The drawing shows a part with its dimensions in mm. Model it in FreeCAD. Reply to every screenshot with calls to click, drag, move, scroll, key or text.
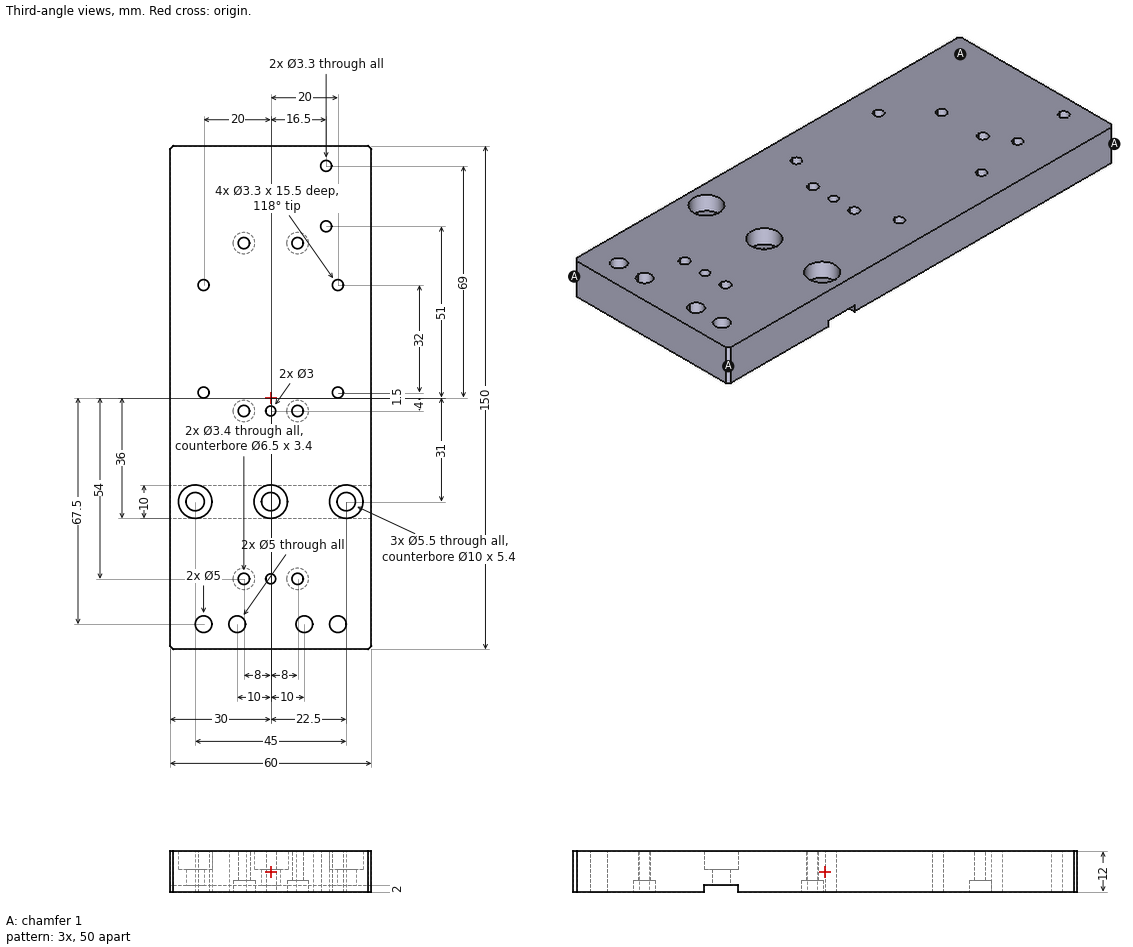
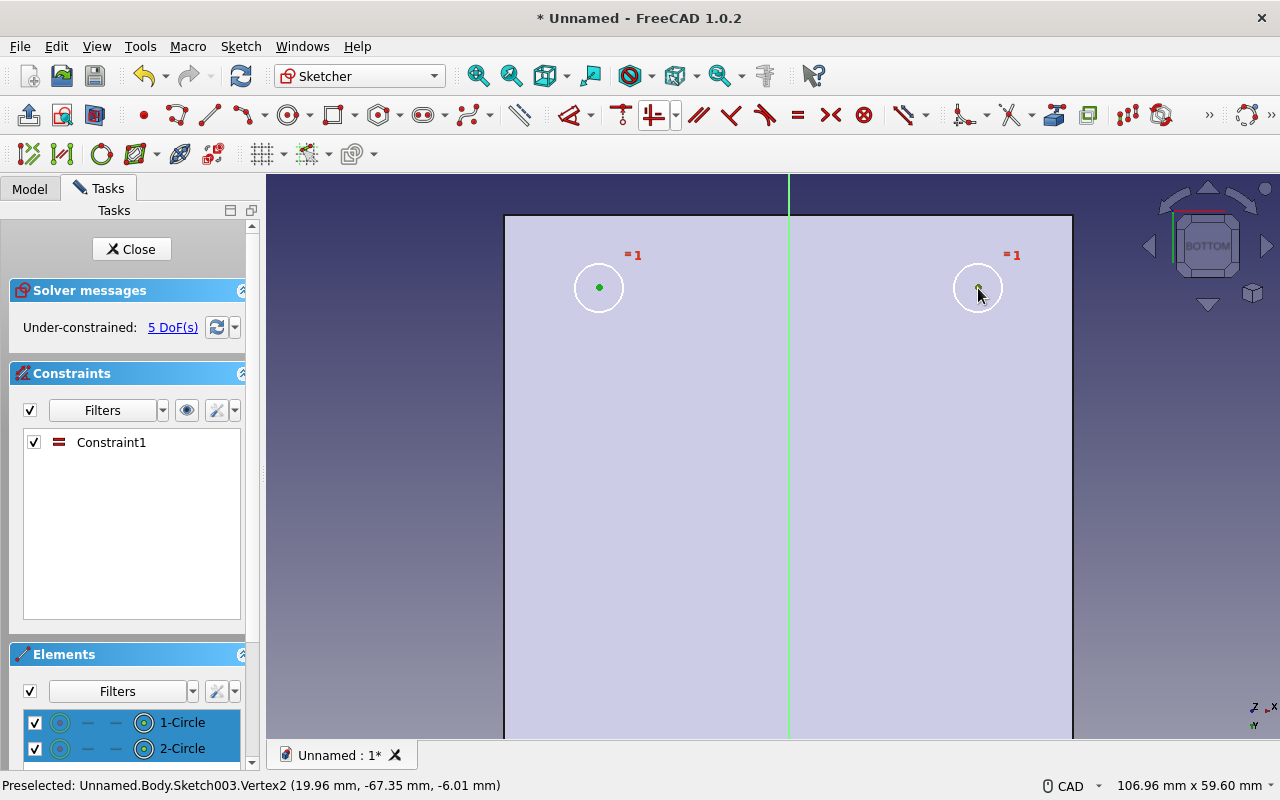
click(676, 116)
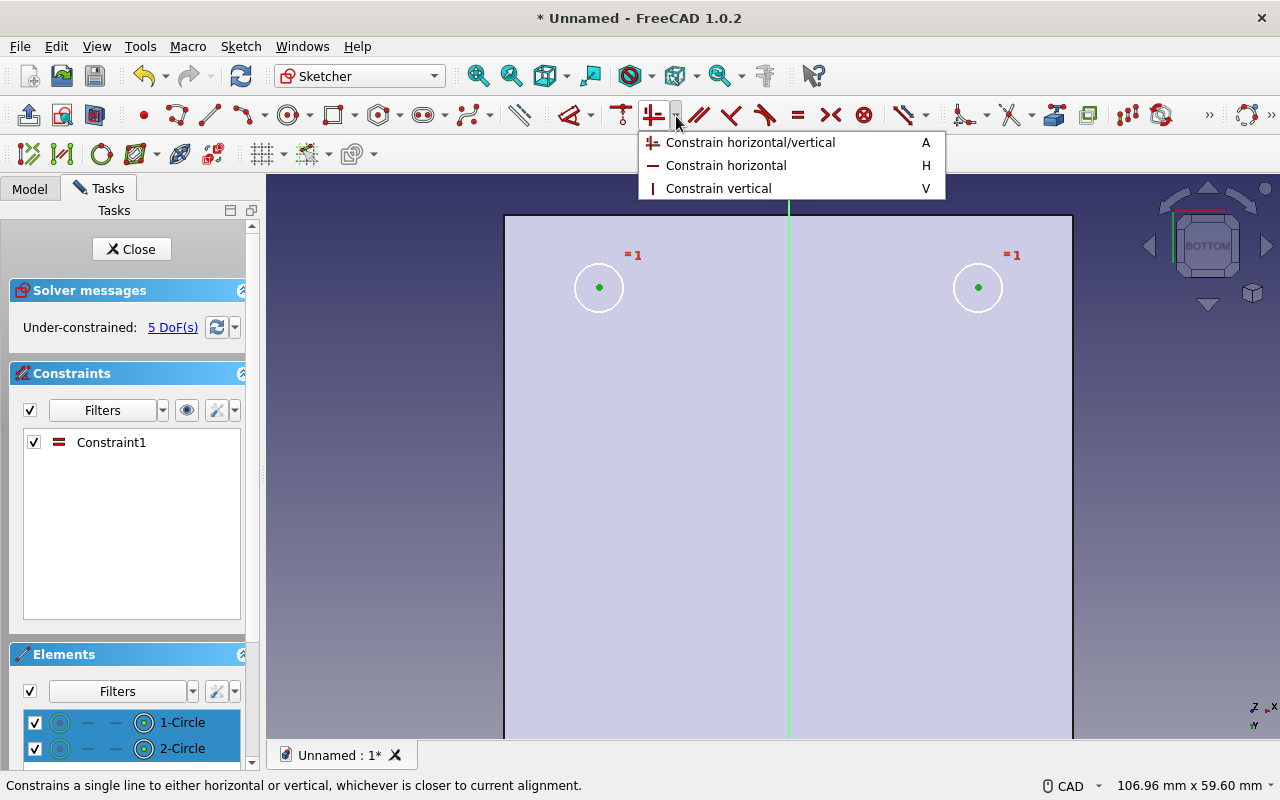
click(792, 166)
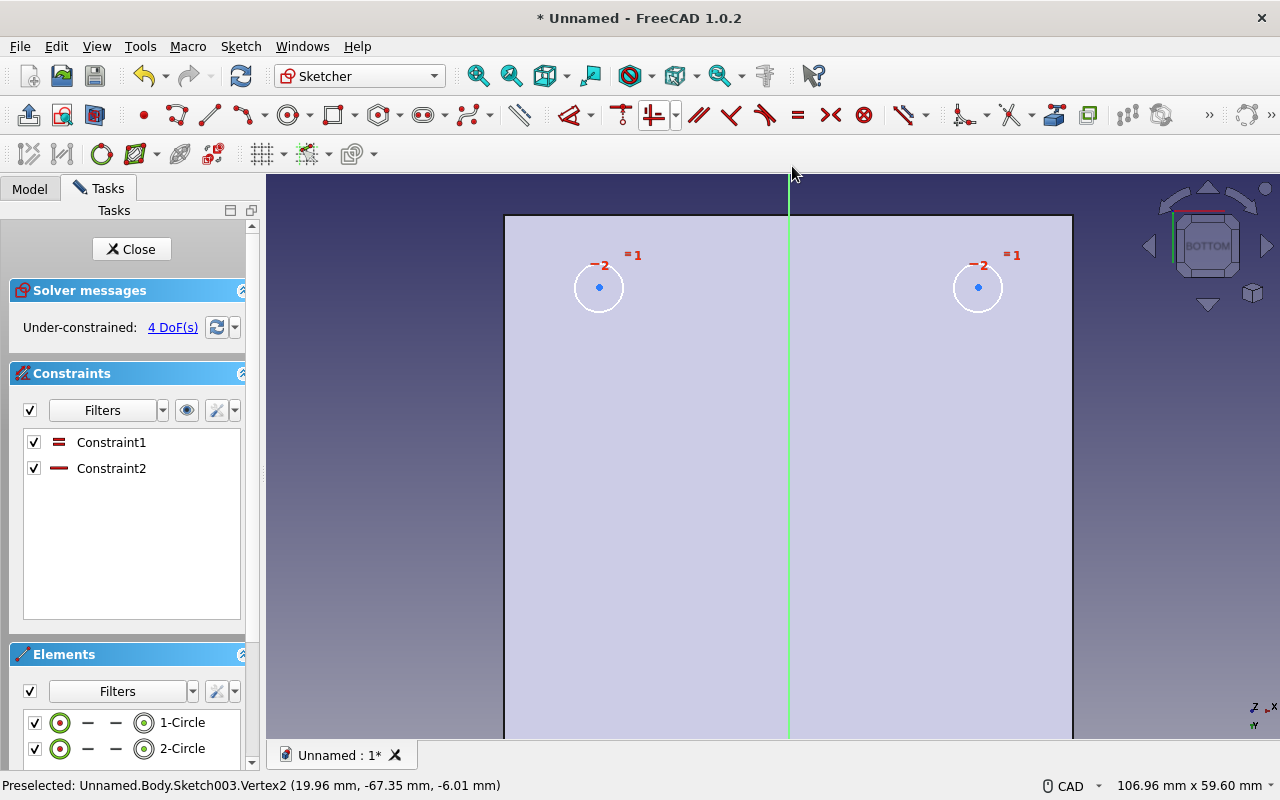
click(568, 116)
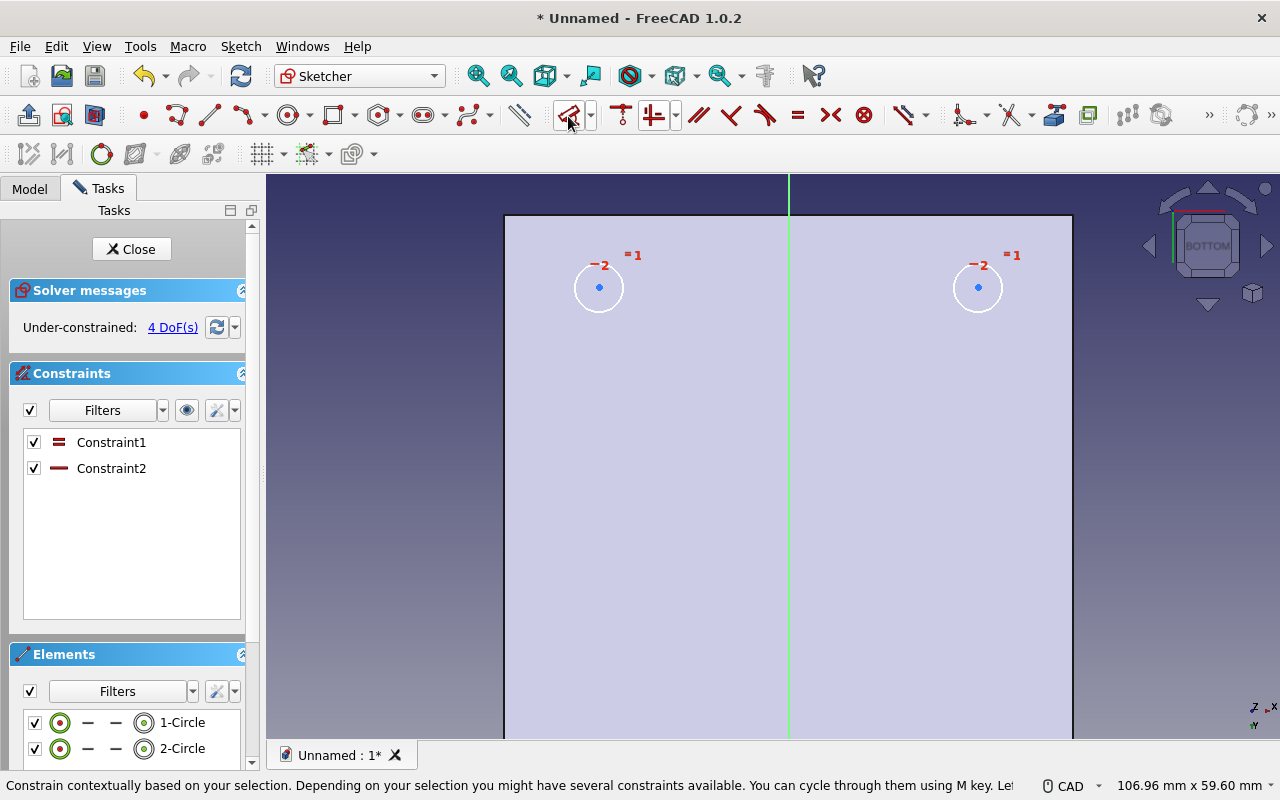
click(616, 271)
click(639, 248)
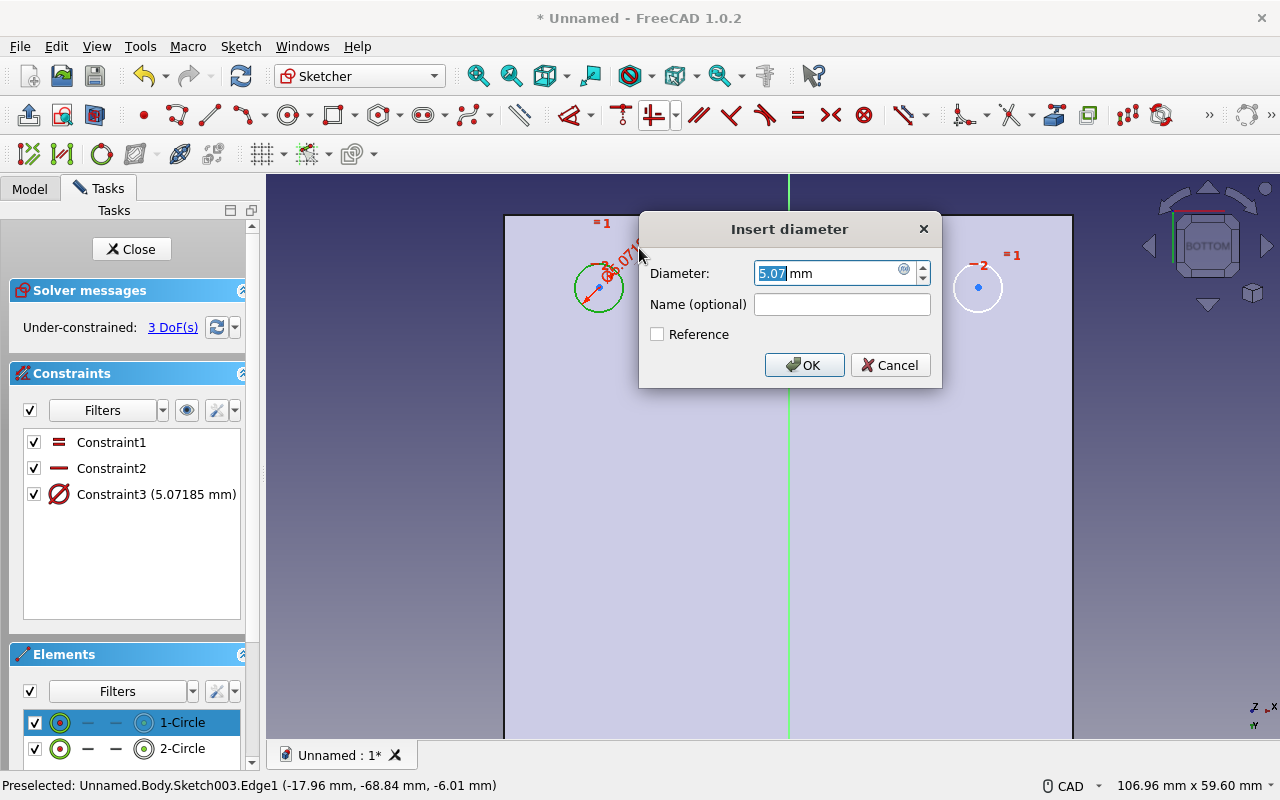
text(5)
key(Return)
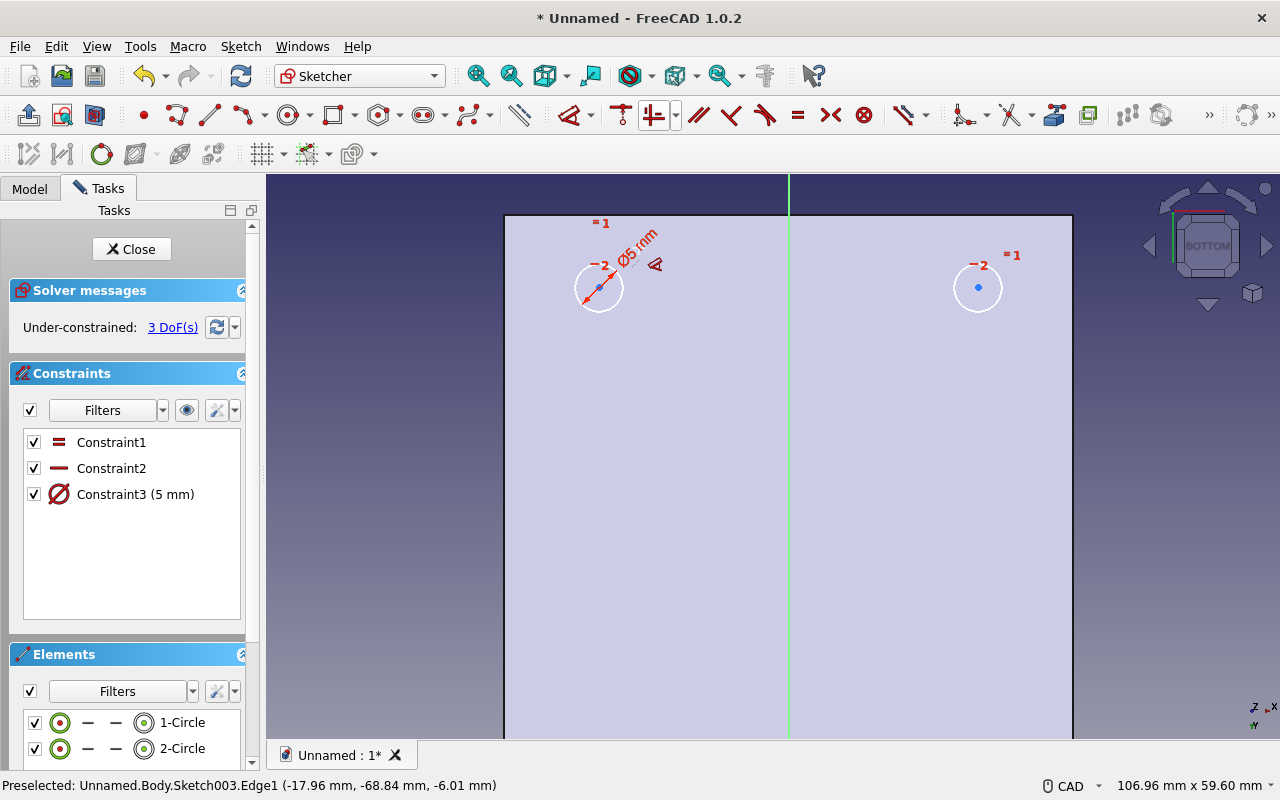
click(599, 288)
click(738, 254)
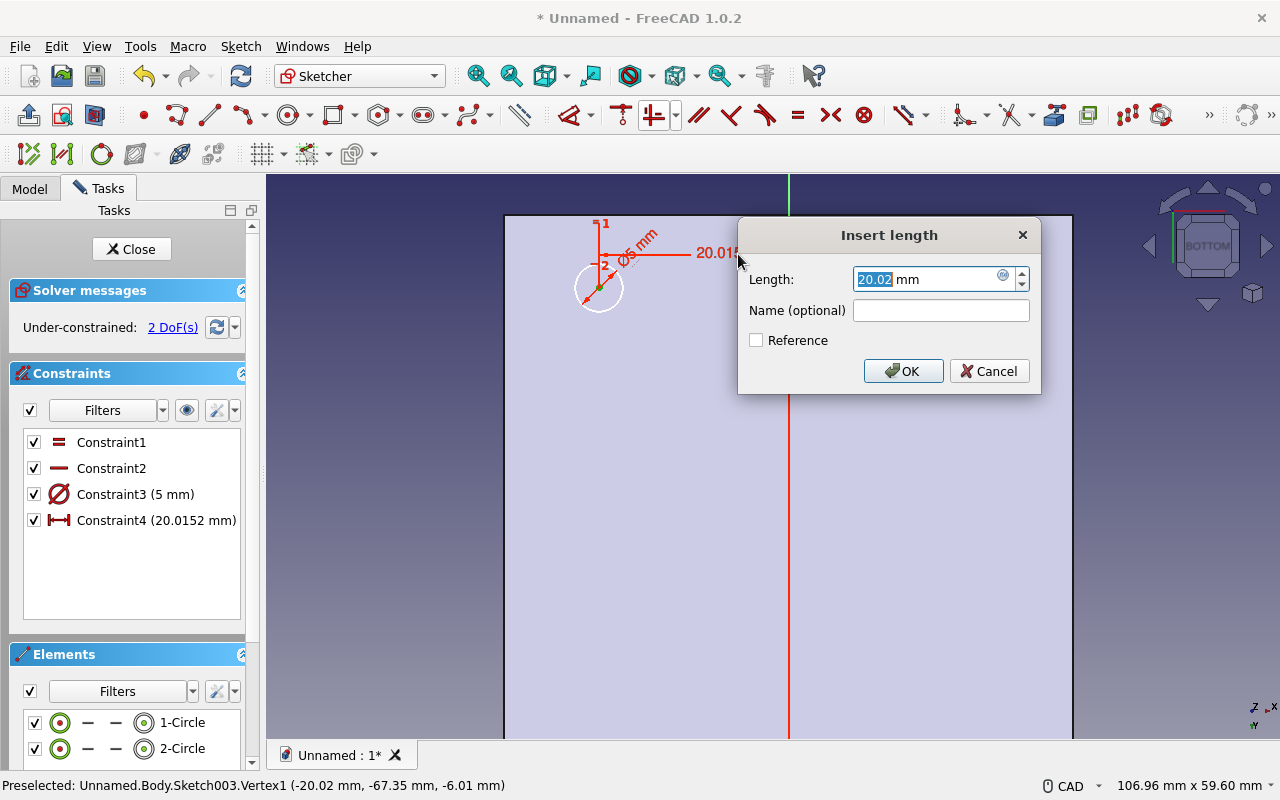
text(20)
key(Return)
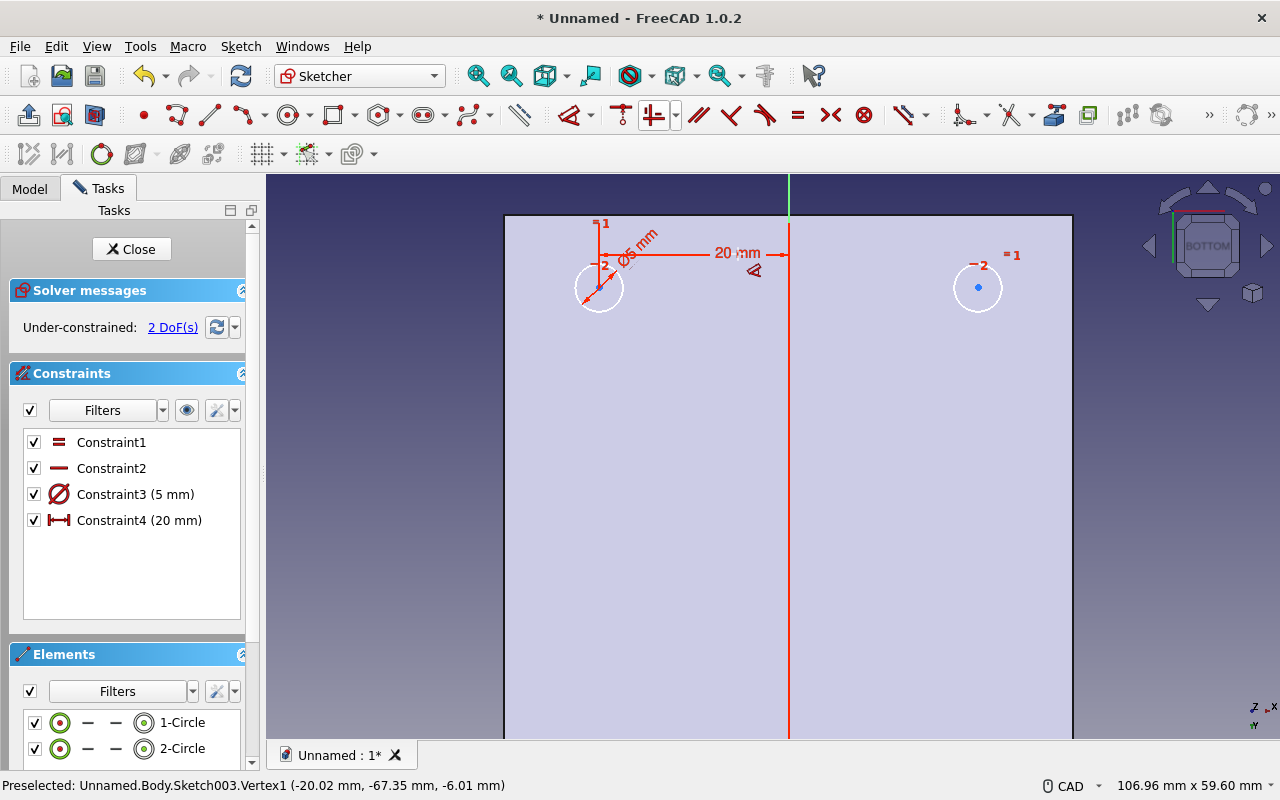
click(978, 288)
click(883, 254)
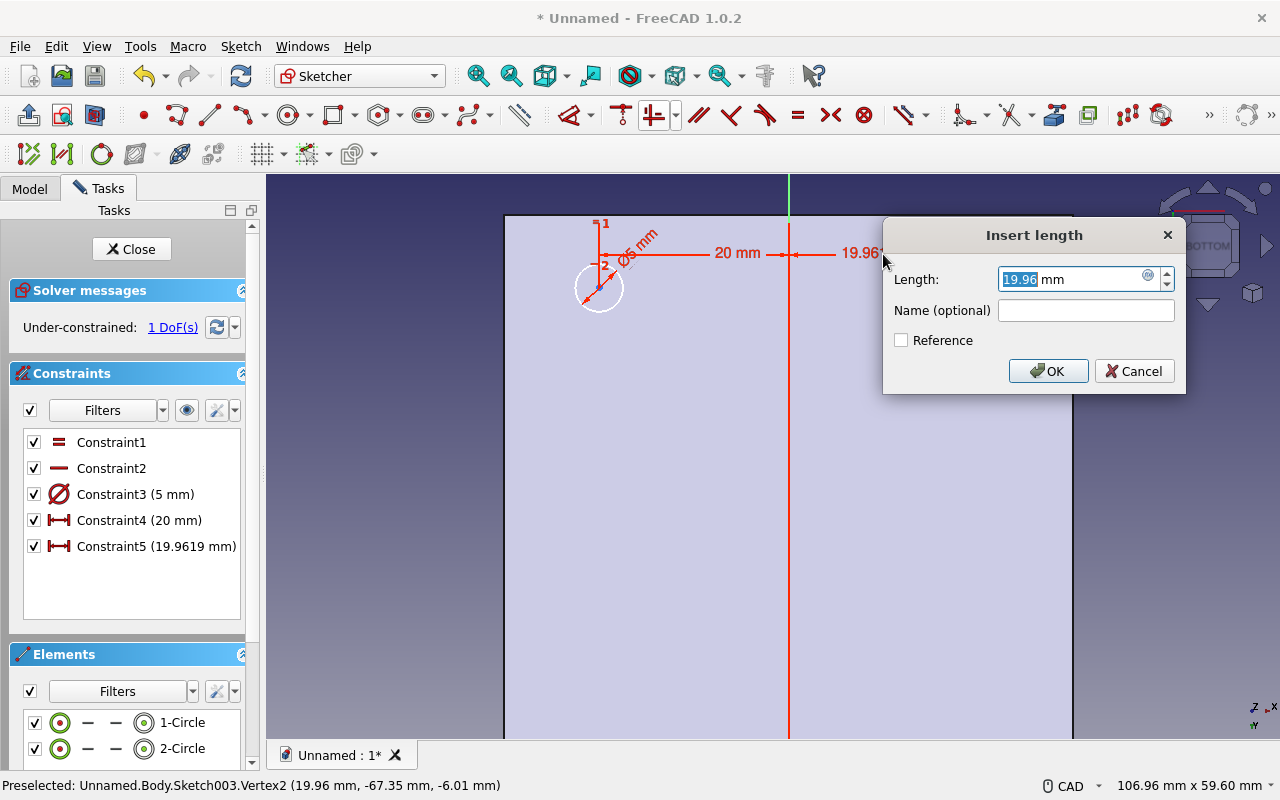
text(20)
key(Return)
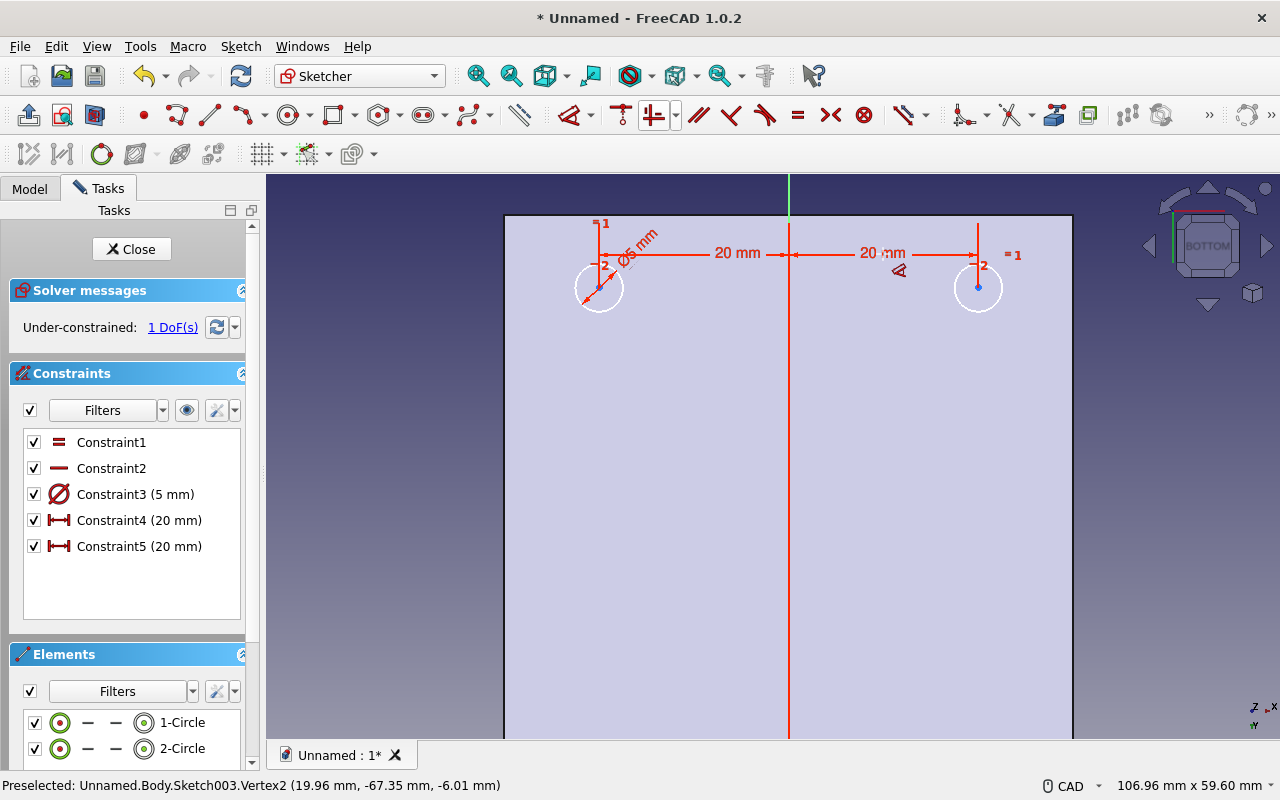
click(599, 288)
click(565, 500)